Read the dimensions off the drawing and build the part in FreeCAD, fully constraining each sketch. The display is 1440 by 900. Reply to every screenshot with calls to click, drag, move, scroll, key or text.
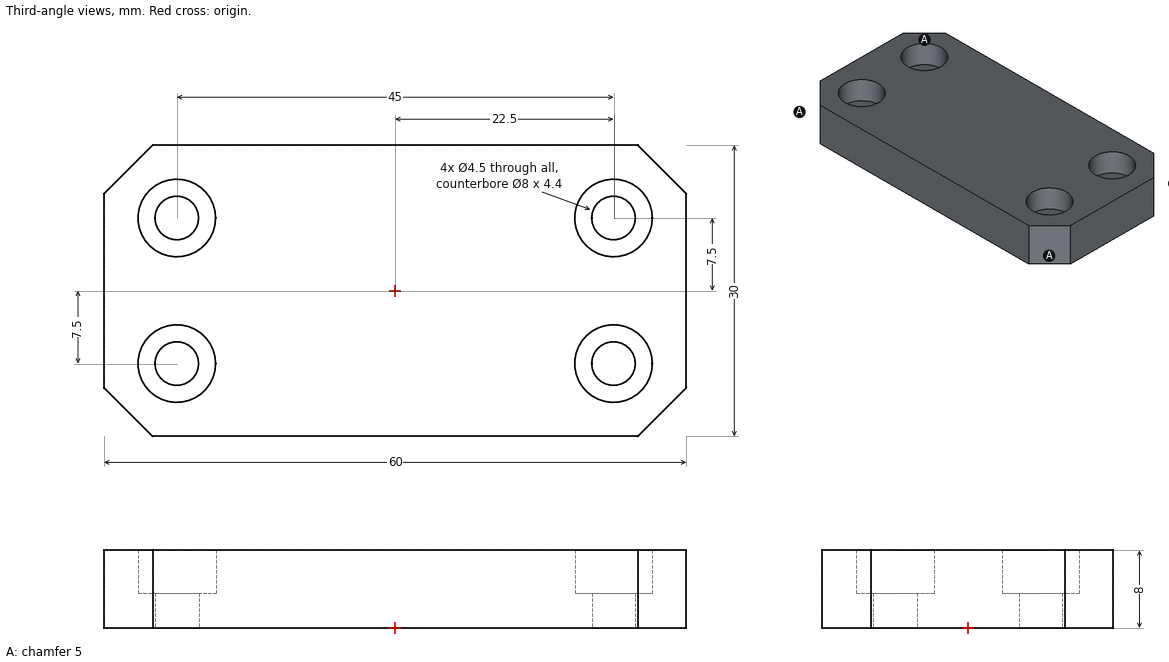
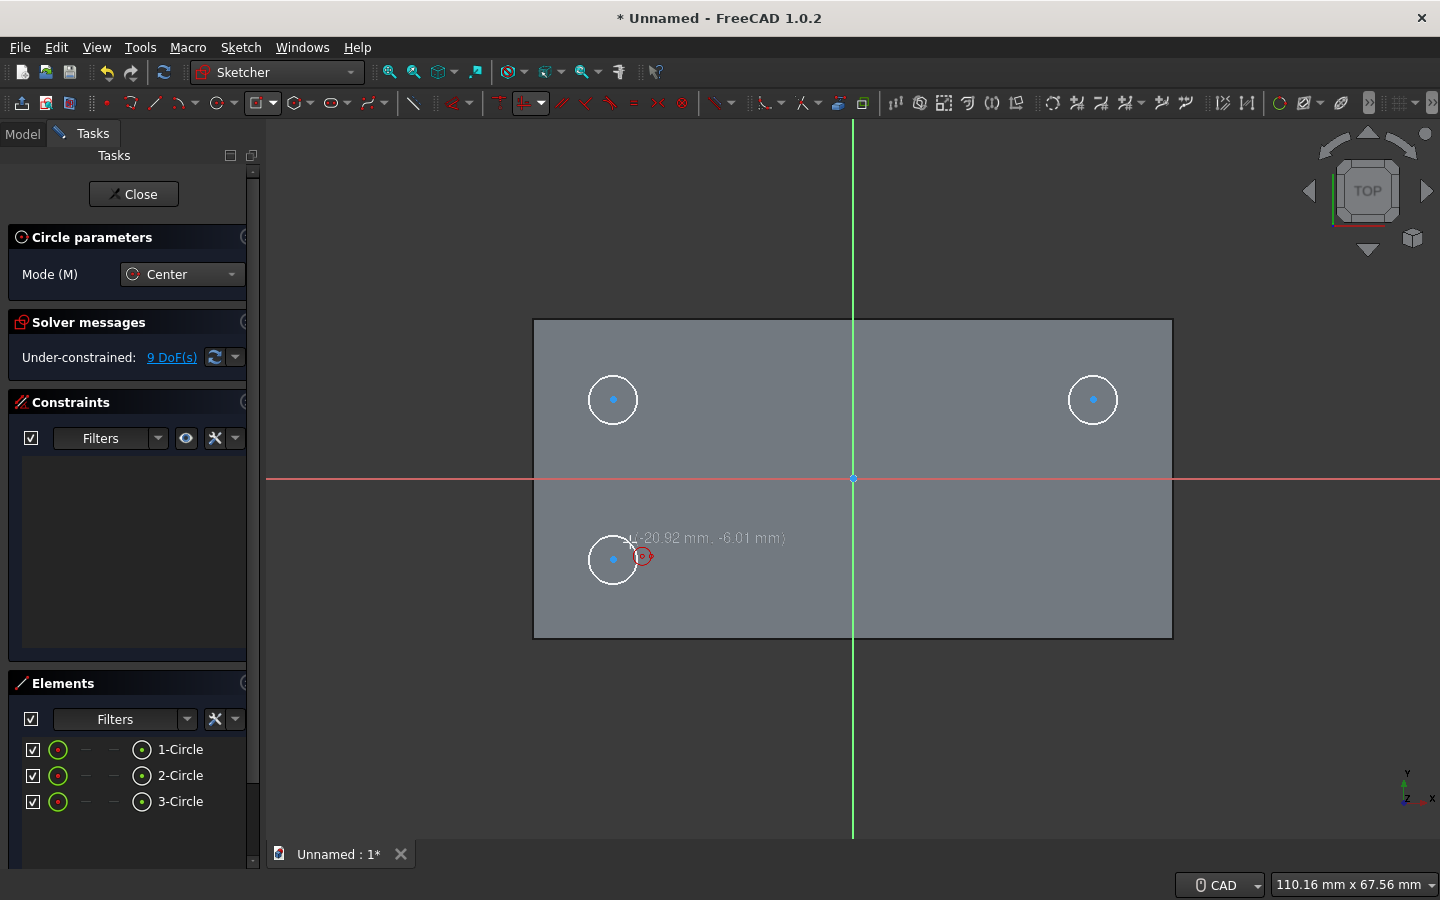
click(1093, 559)
click(1110, 542)
key(Escape)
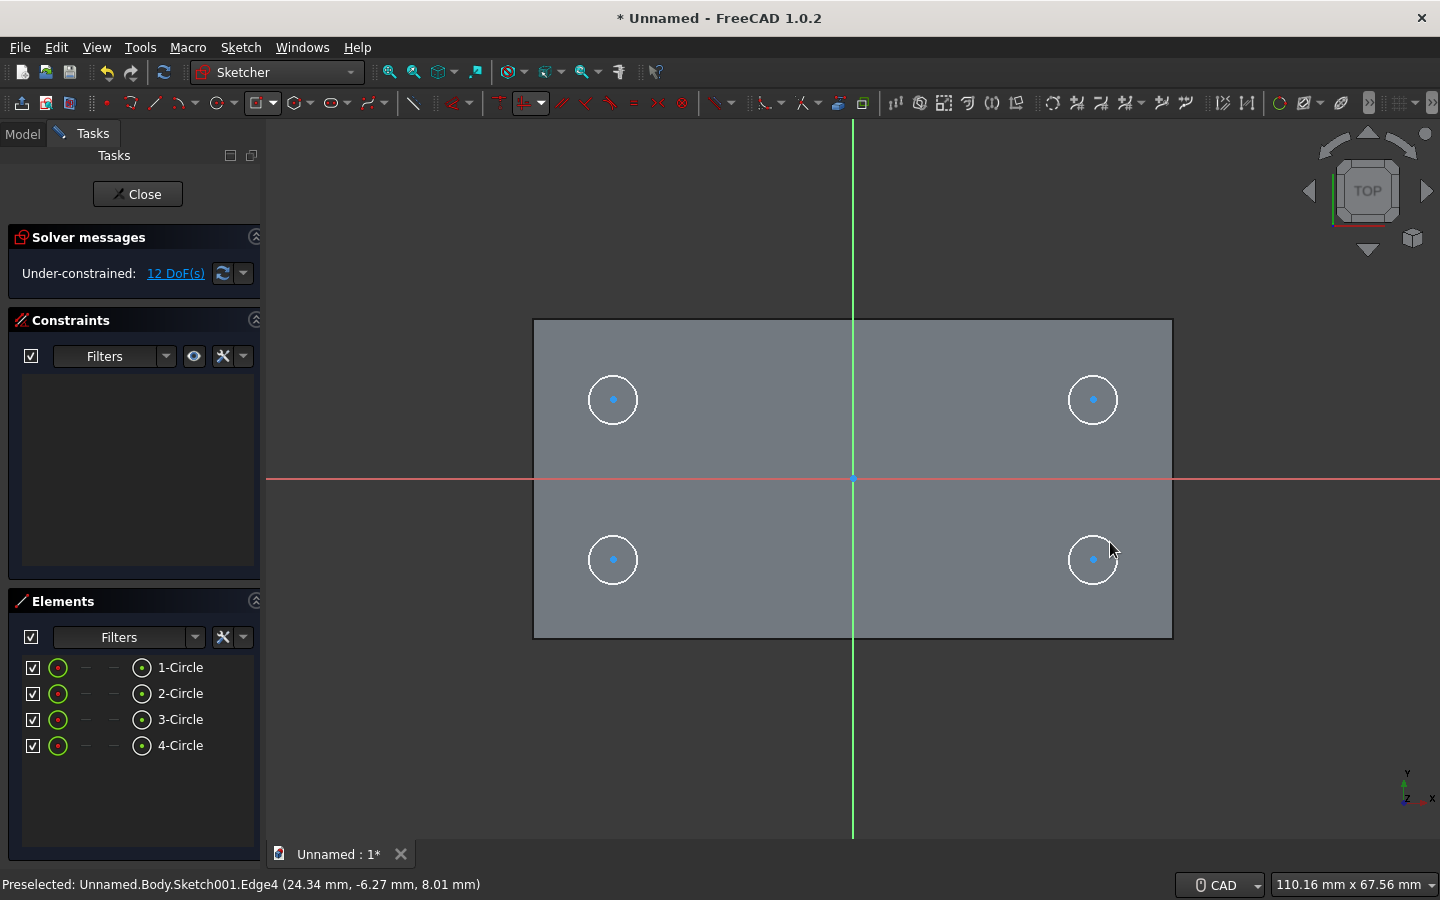
click(1110, 383)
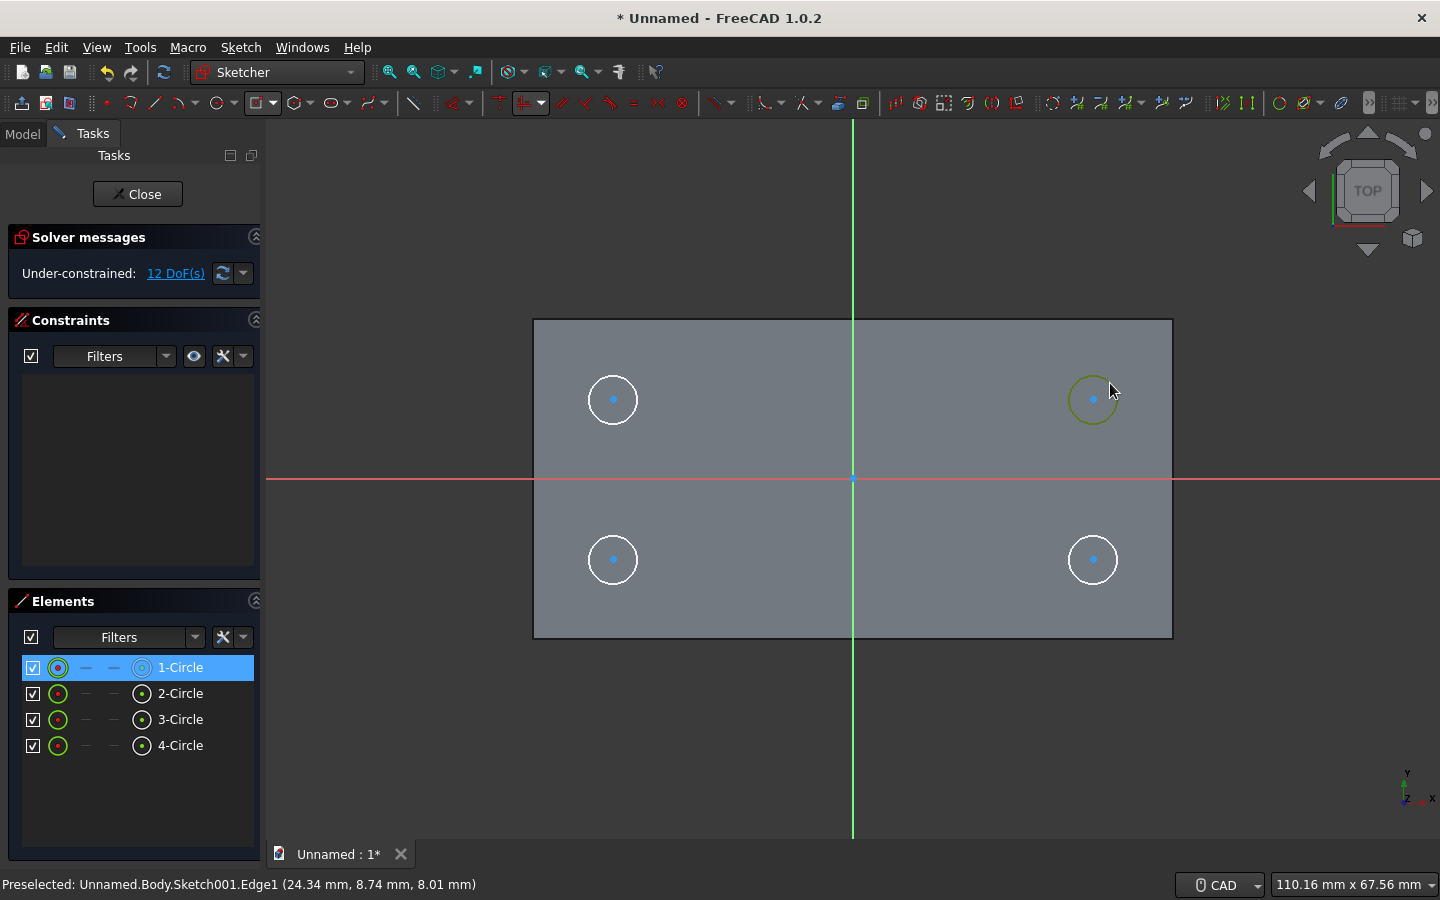
click(630, 383)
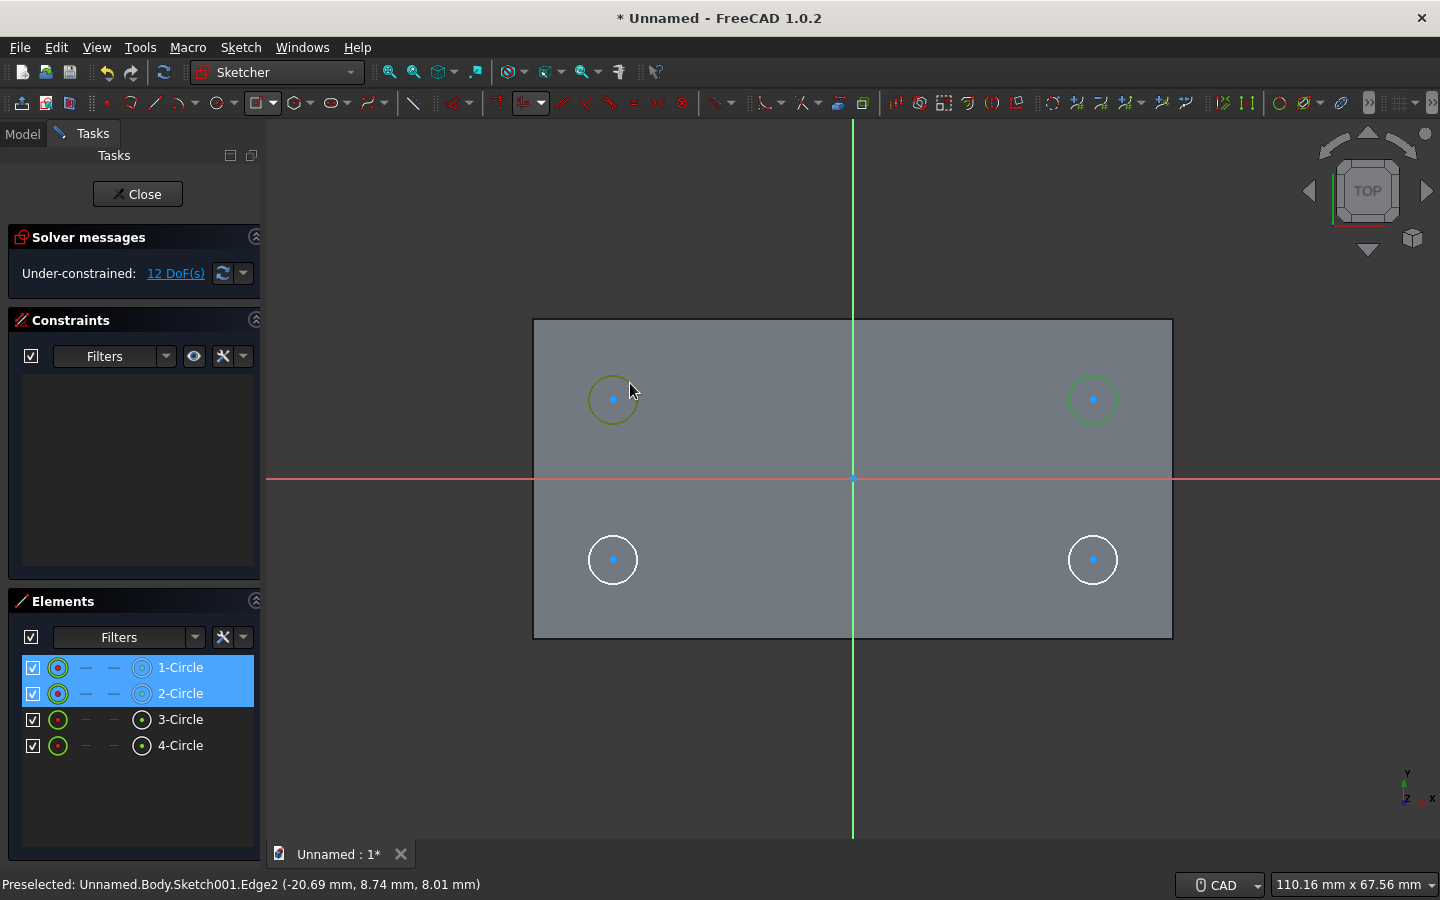
click(630, 543)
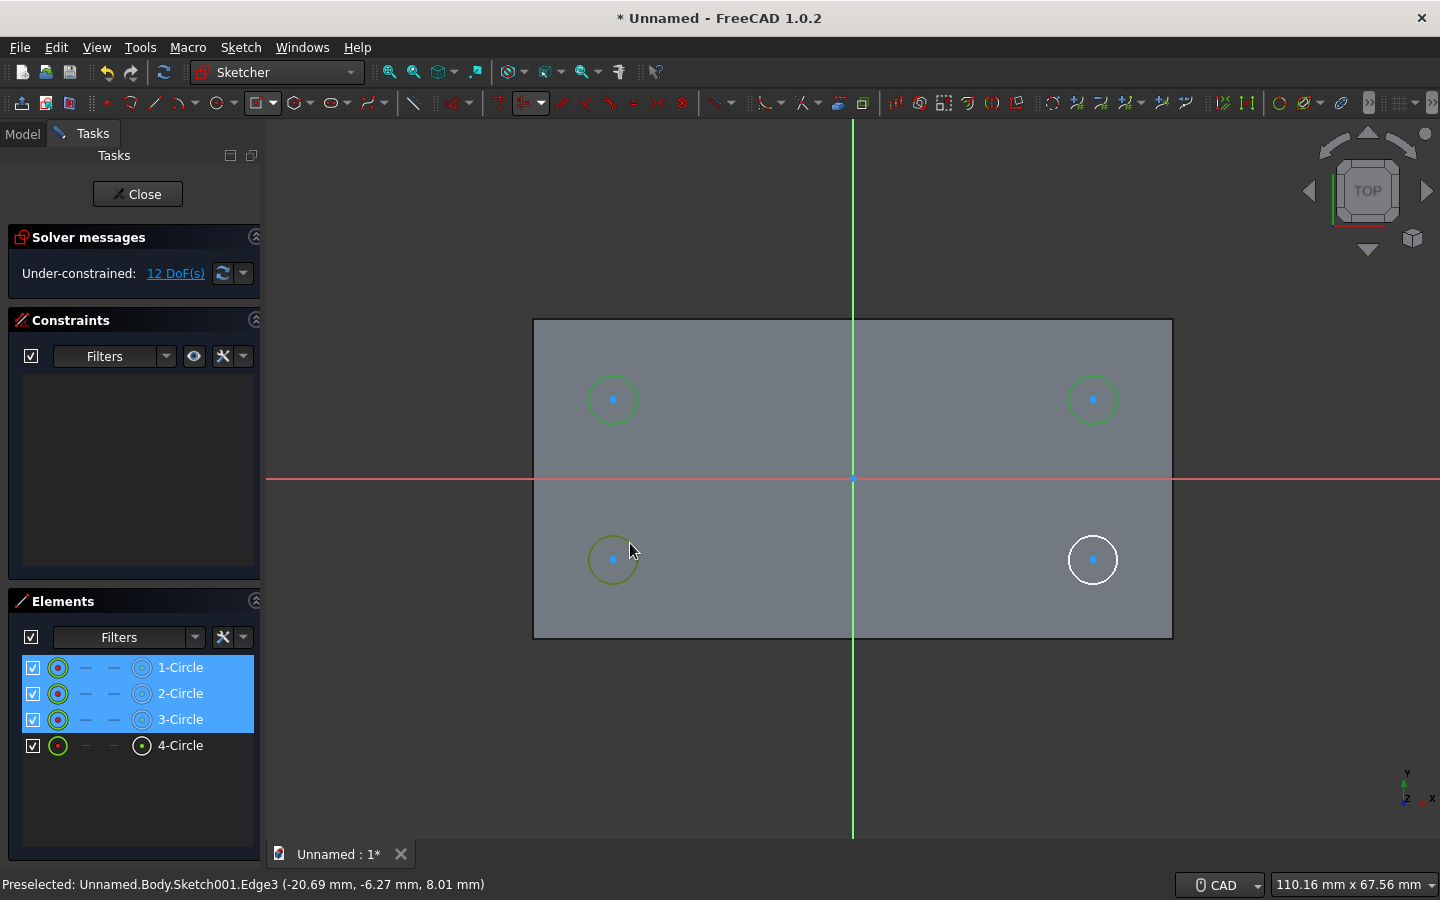
click(1110, 543)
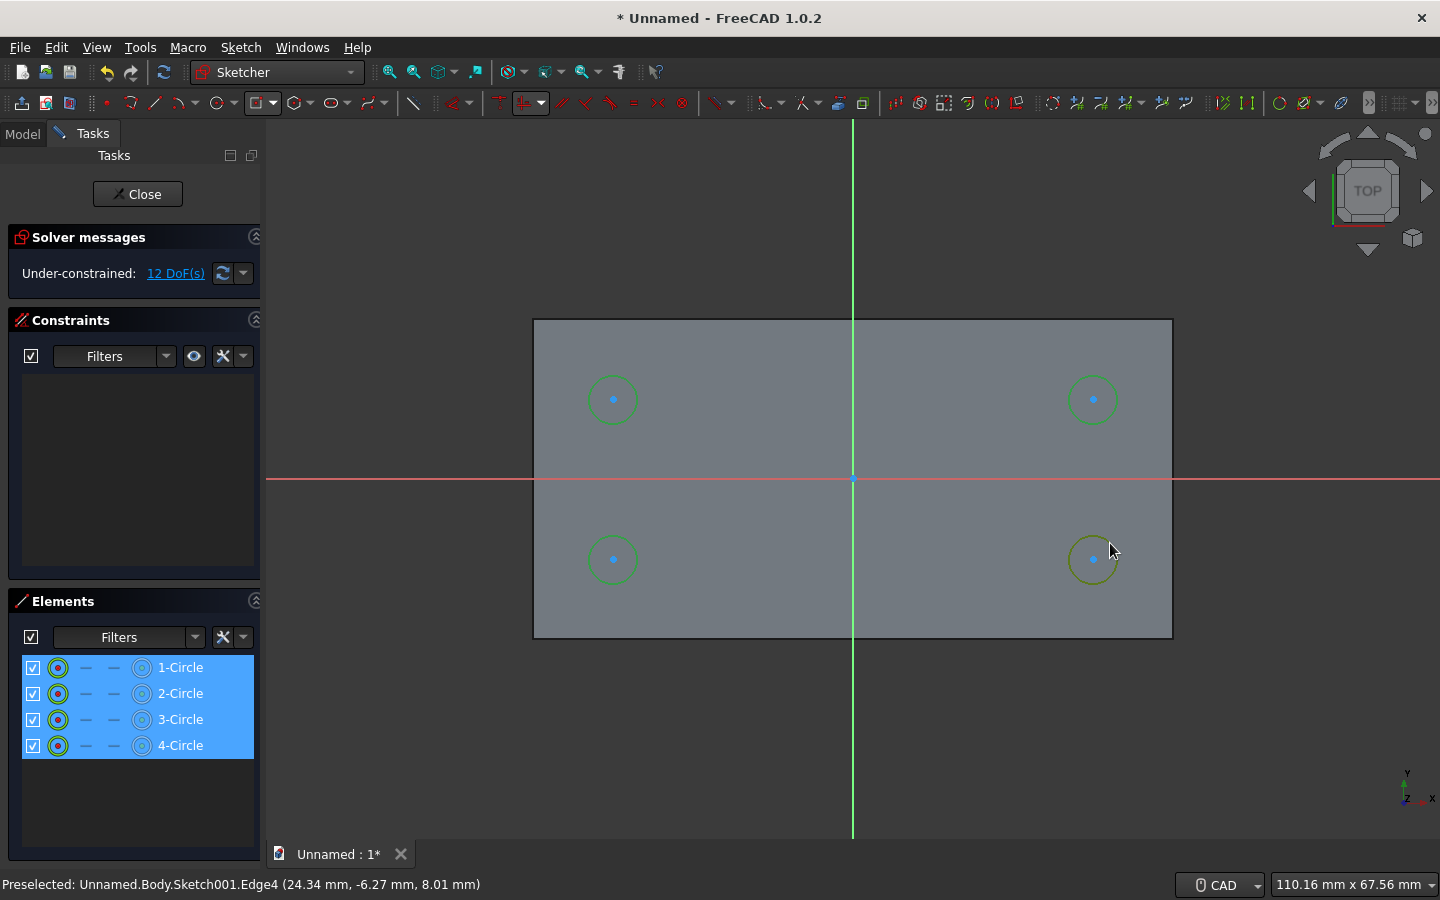
click(634, 104)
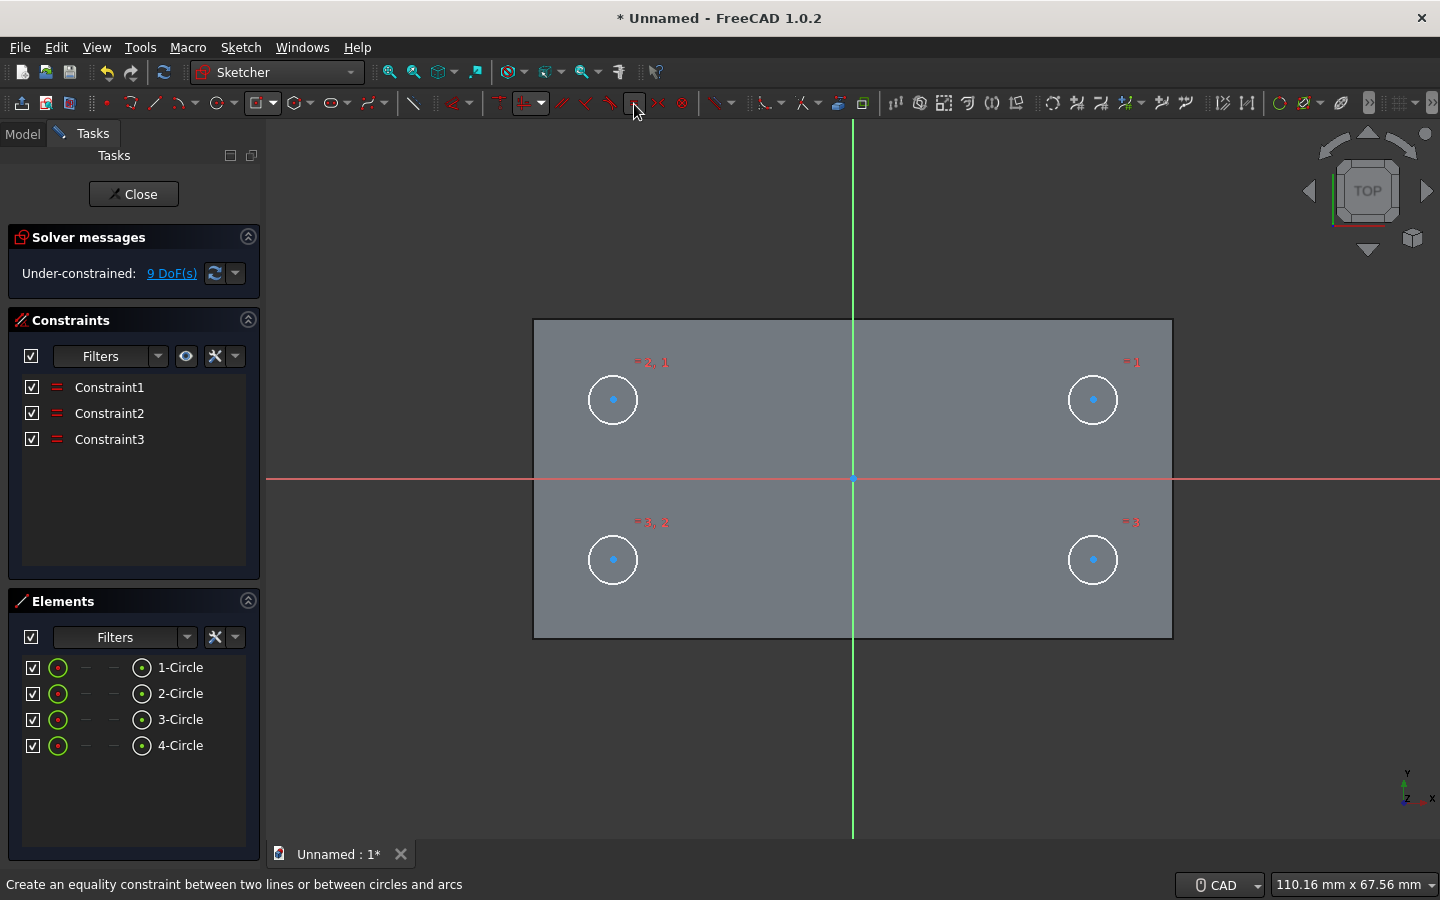
click(1093, 400)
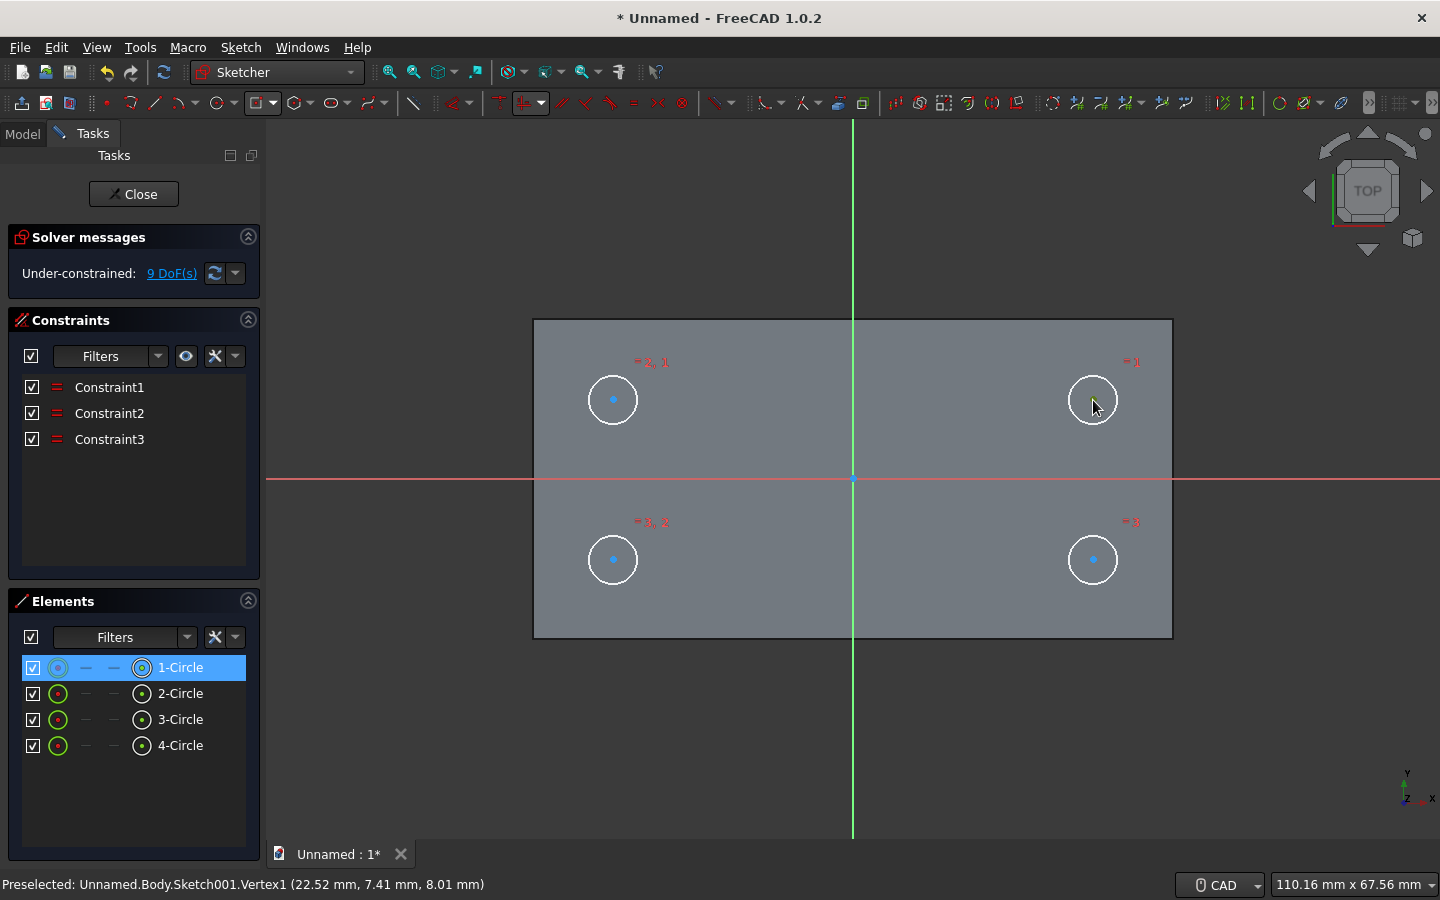
click(613, 400)